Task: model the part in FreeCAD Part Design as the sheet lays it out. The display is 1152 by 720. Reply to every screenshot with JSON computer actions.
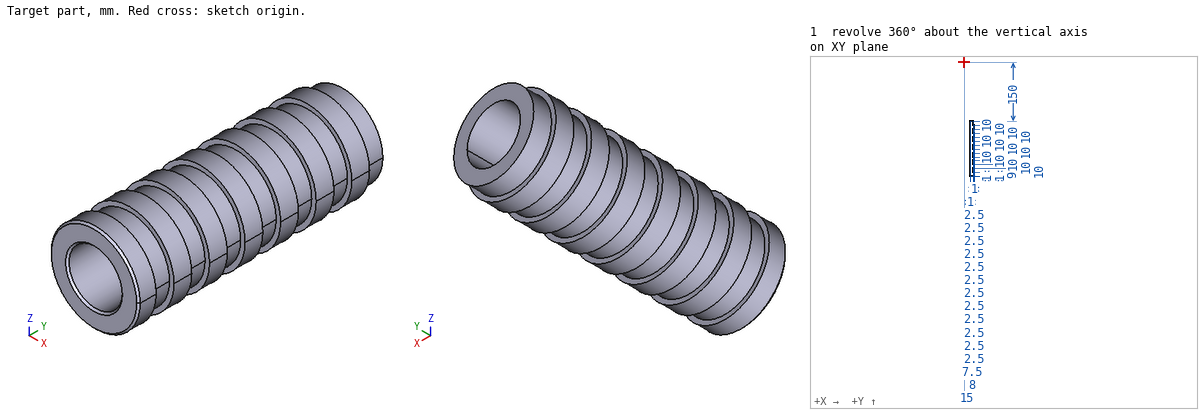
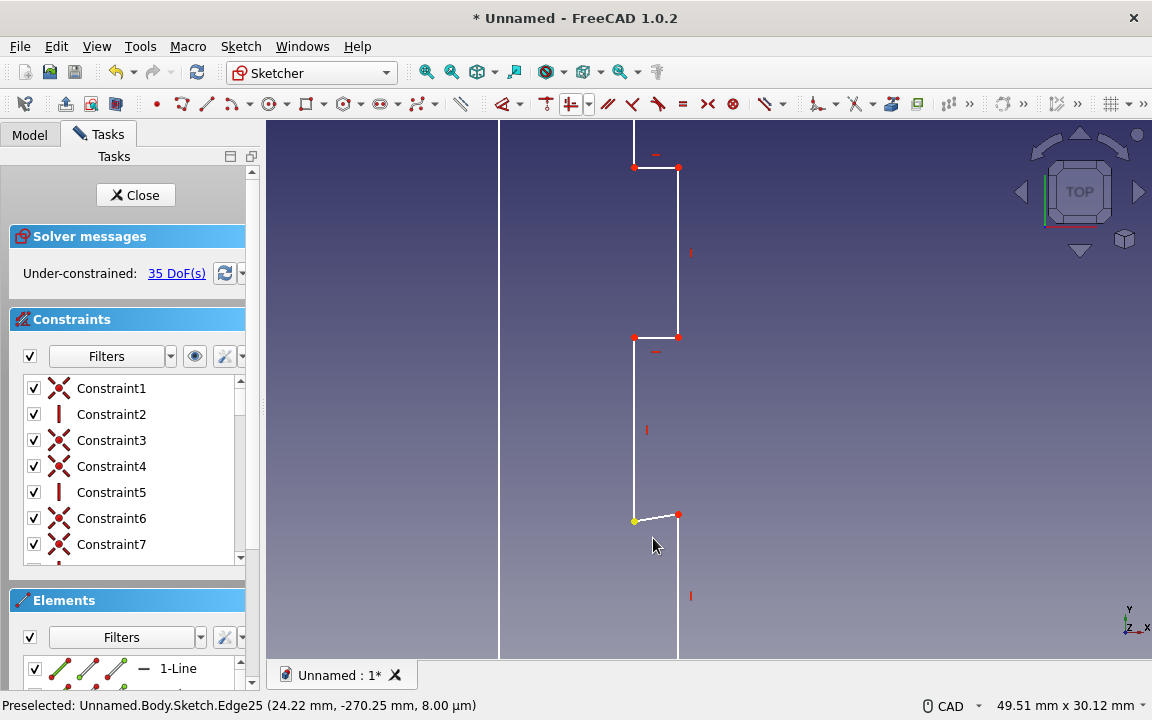
{"action": "left_click", "coordinate": [647, 519]}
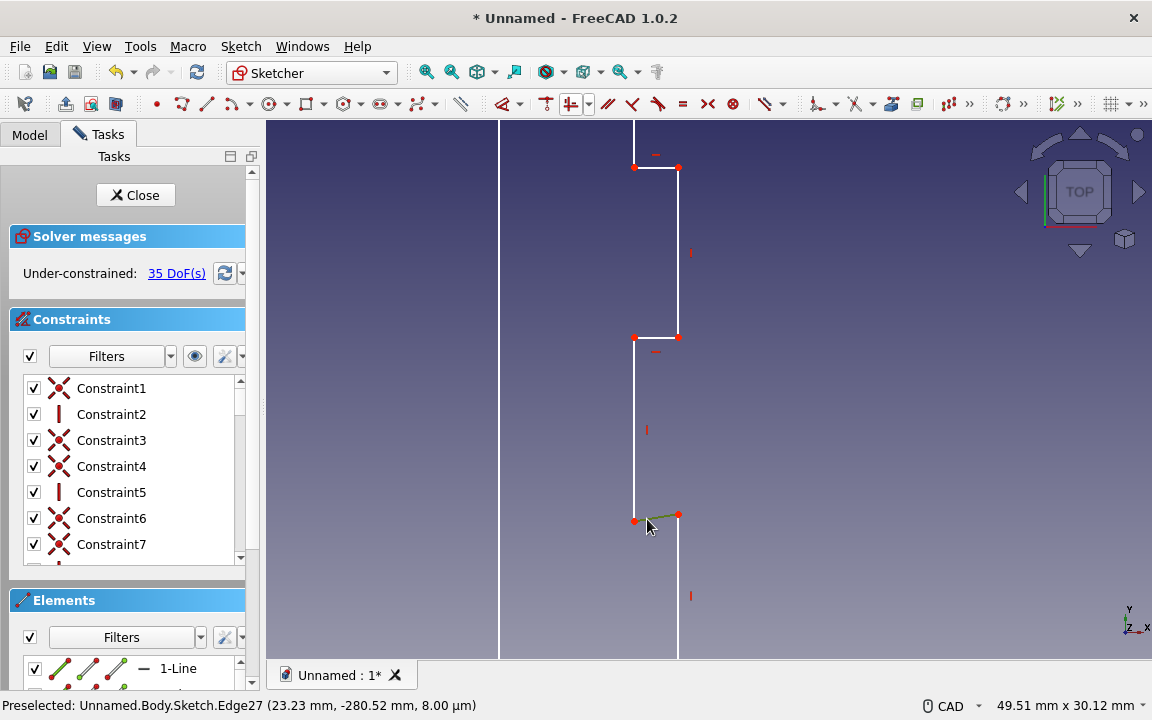
{"action": "key", "text": "h"}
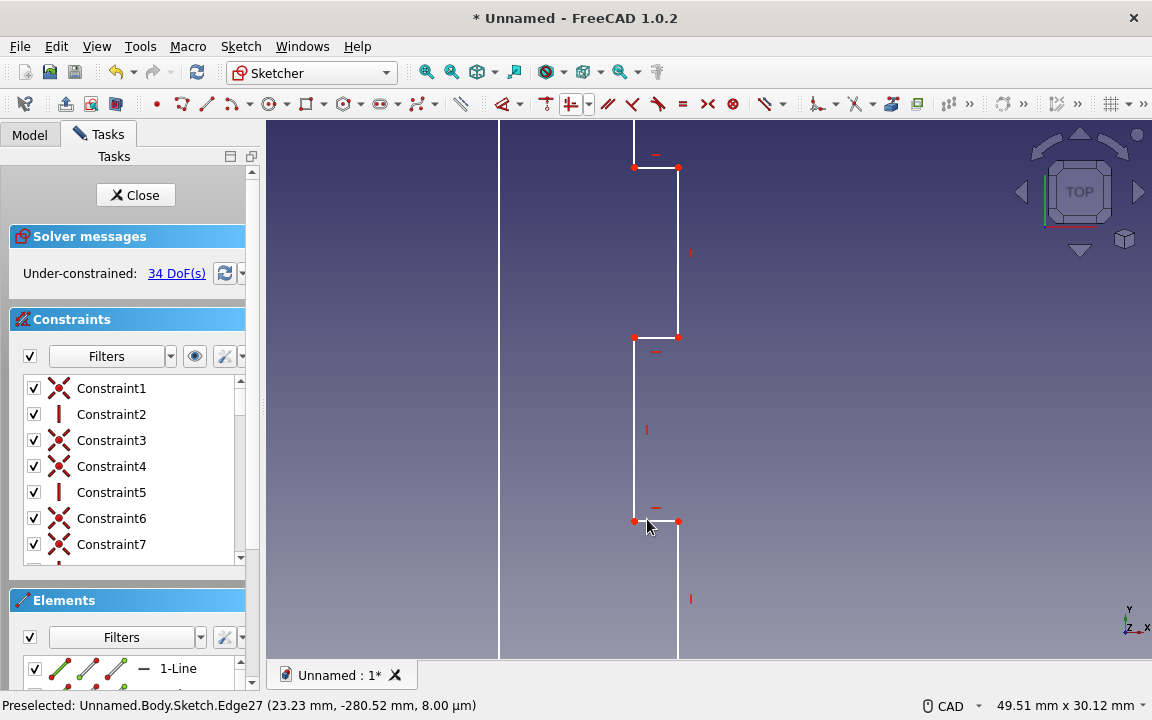
{"action": "key", "text": "d"}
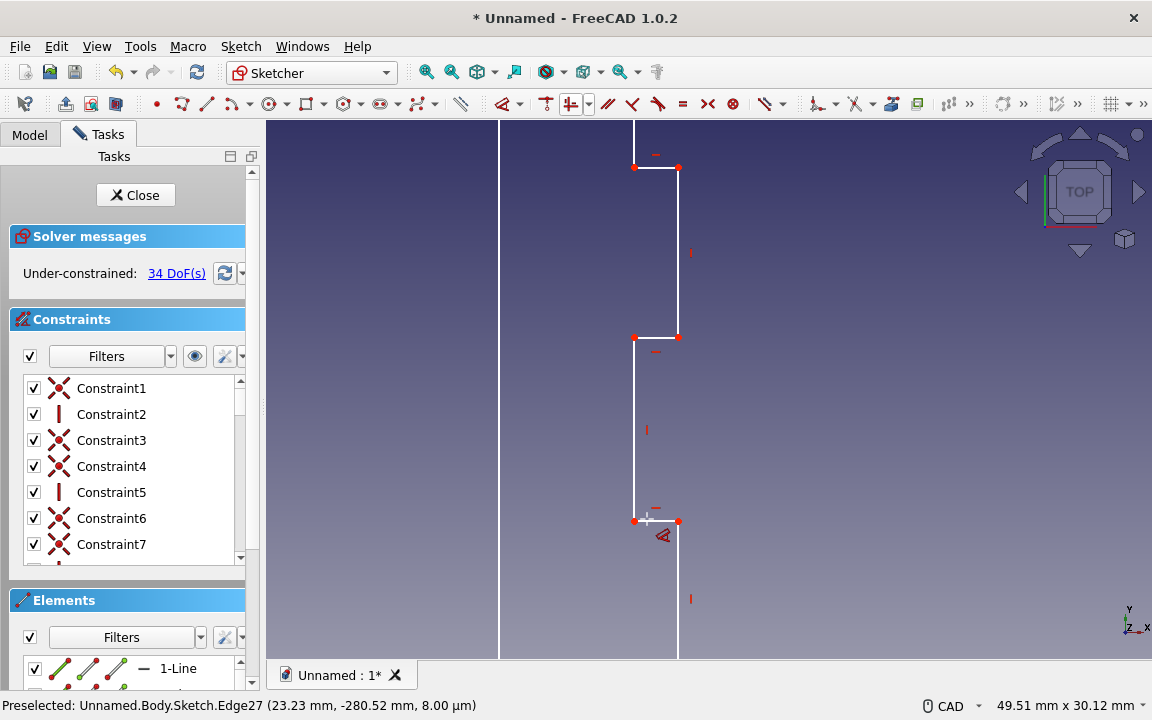
{"action": "scroll", "coordinate": [653, 538], "scroll_direction": "down", "scroll_amount": 14}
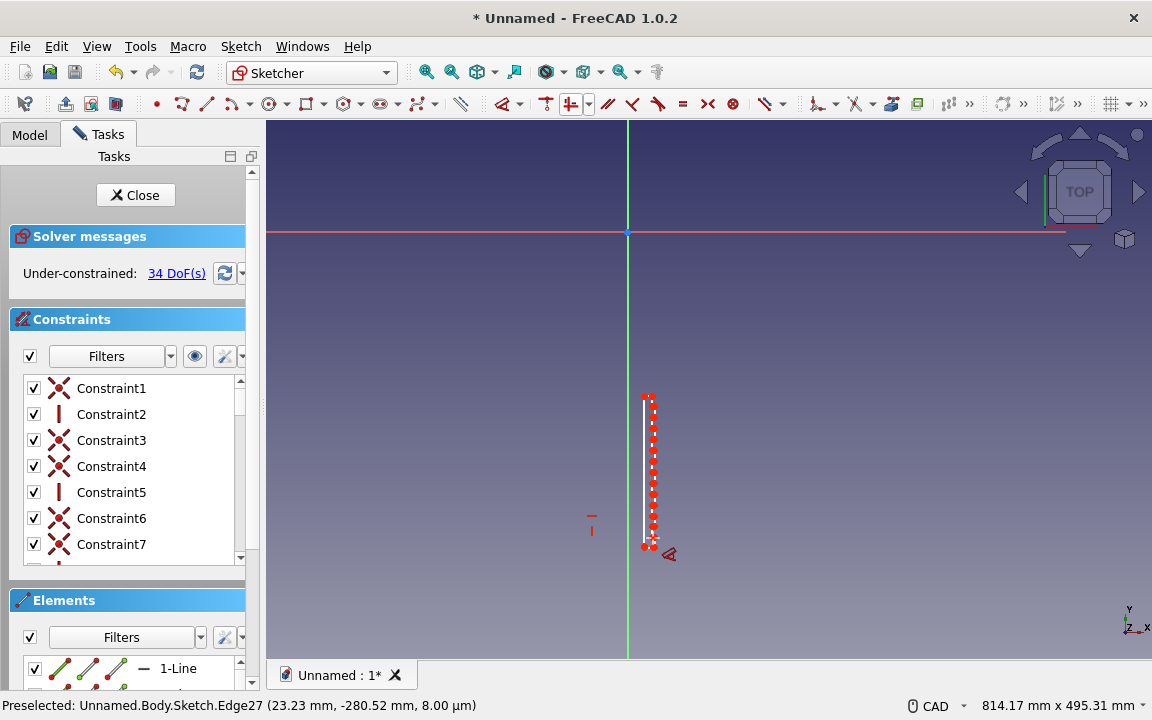
{"action": "scroll", "coordinate": [655, 541], "scroll_direction": "up", "scroll_amount": 8}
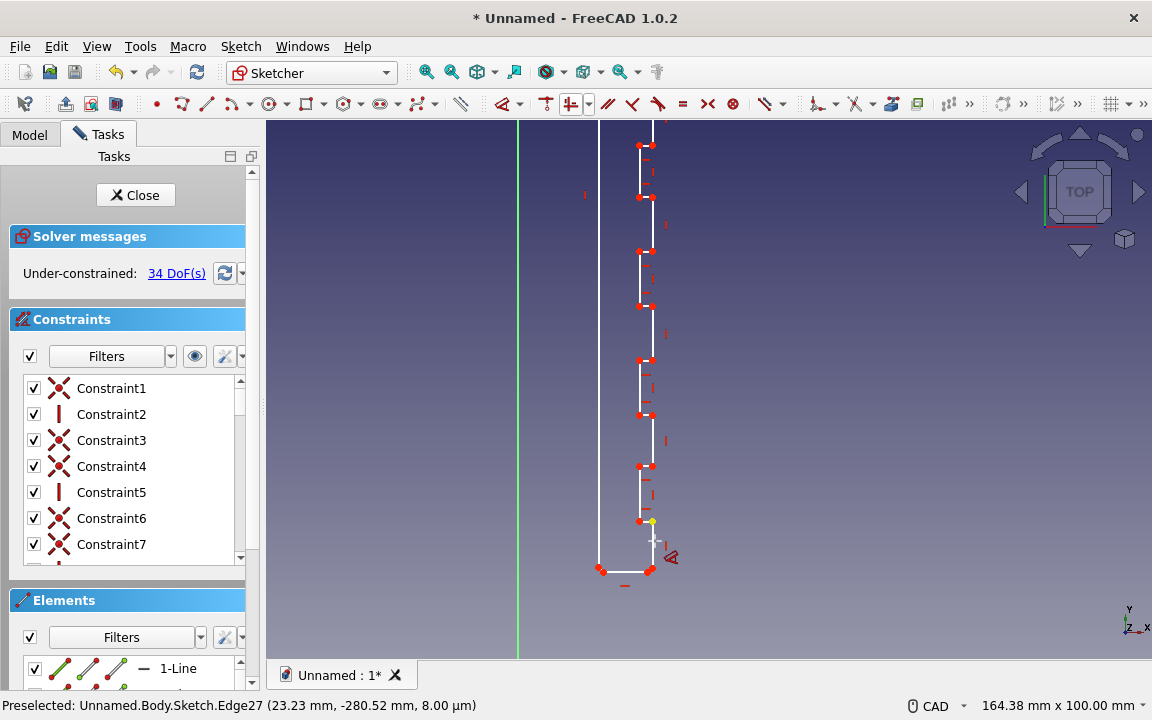
{"action": "left_click", "coordinate": [653, 536]}
{"action": "left_click", "coordinate": [687, 545]}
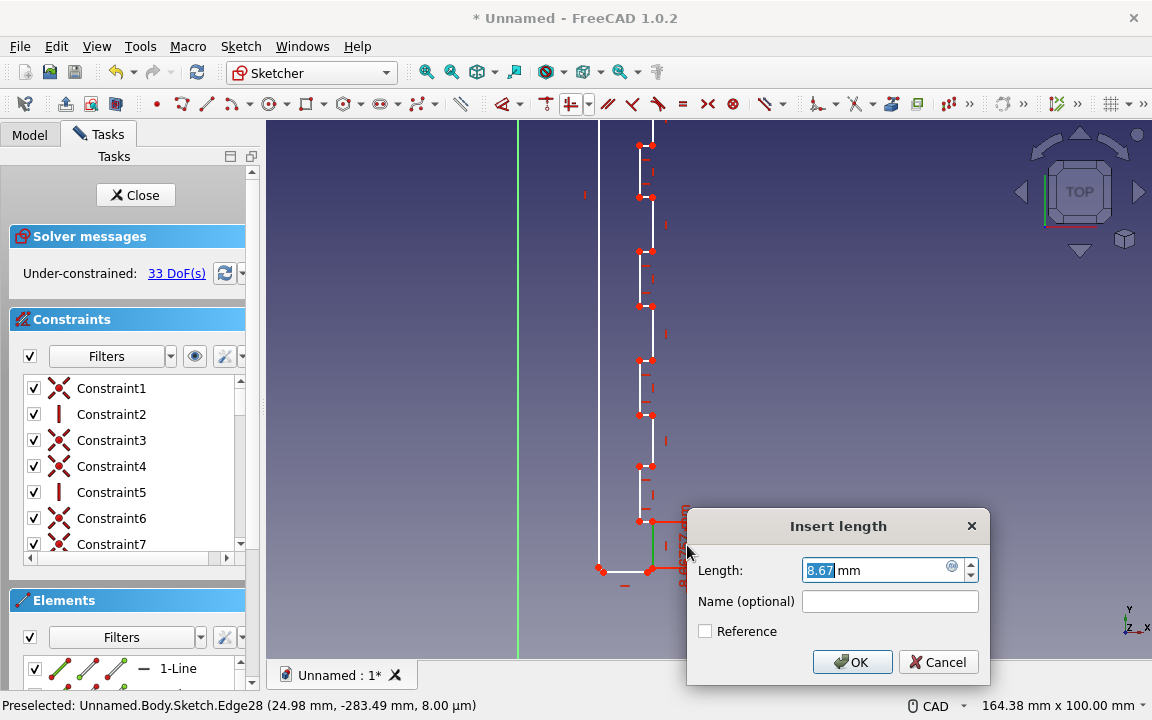
{"action": "type", "text": "9"}
{"action": "key", "text": "Return"}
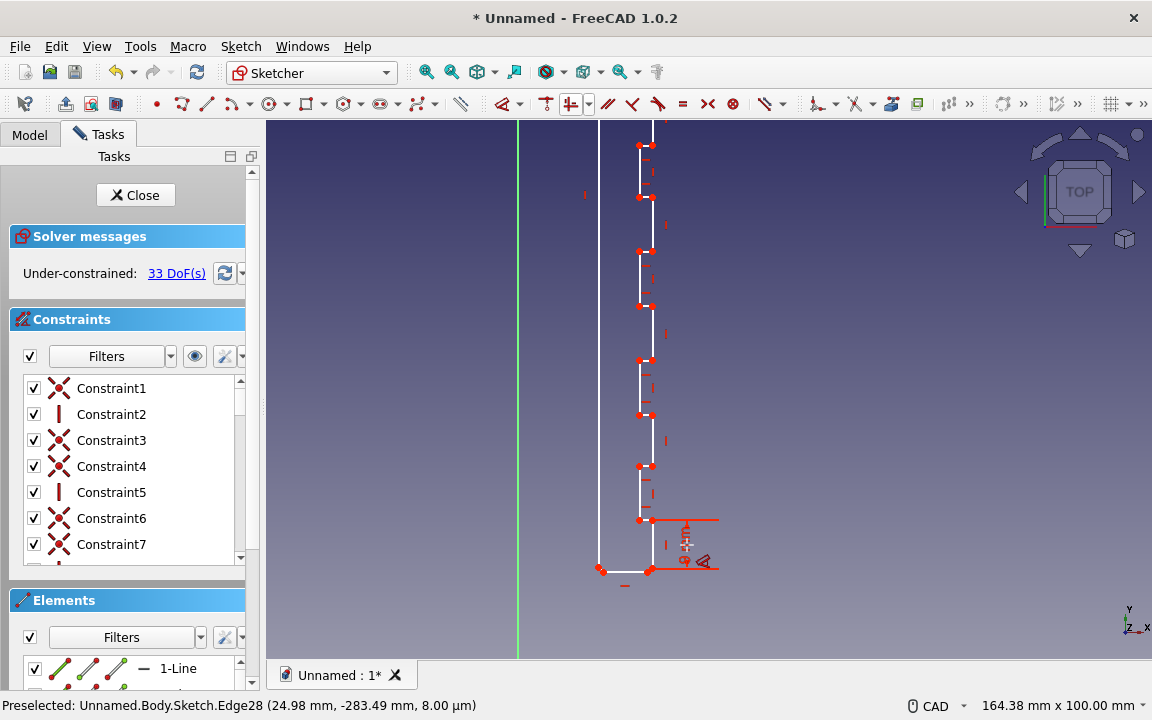
{"action": "left_click", "coordinate": [634, 572]}
{"action": "left_click", "coordinate": [626, 606]}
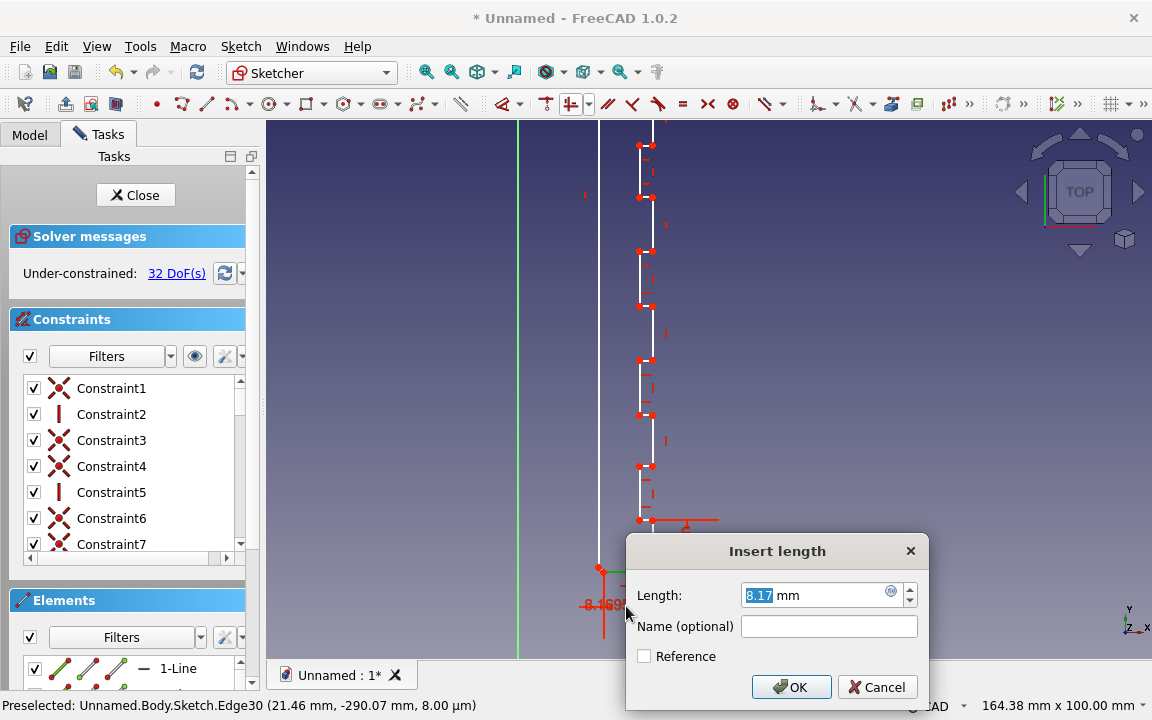
{"action": "type", "text": "8"}
{"action": "key", "text": "Return"}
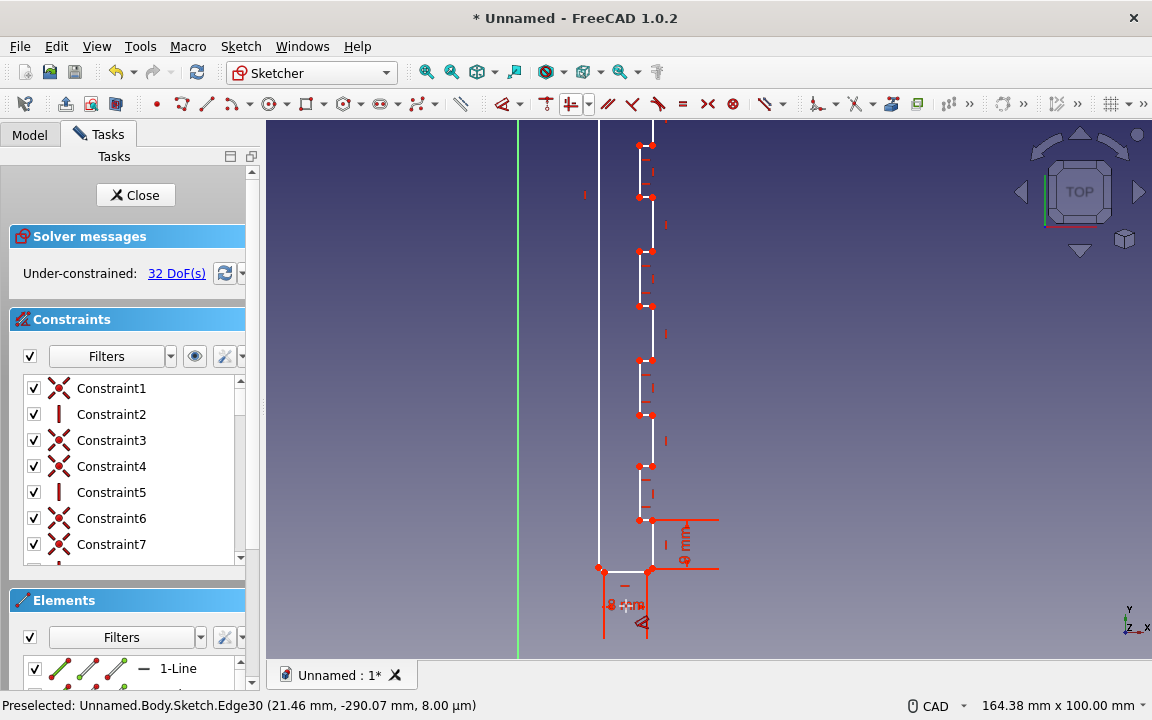
{"action": "scroll", "coordinate": [654, 541], "scroll_direction": "down", "scroll_amount": 8}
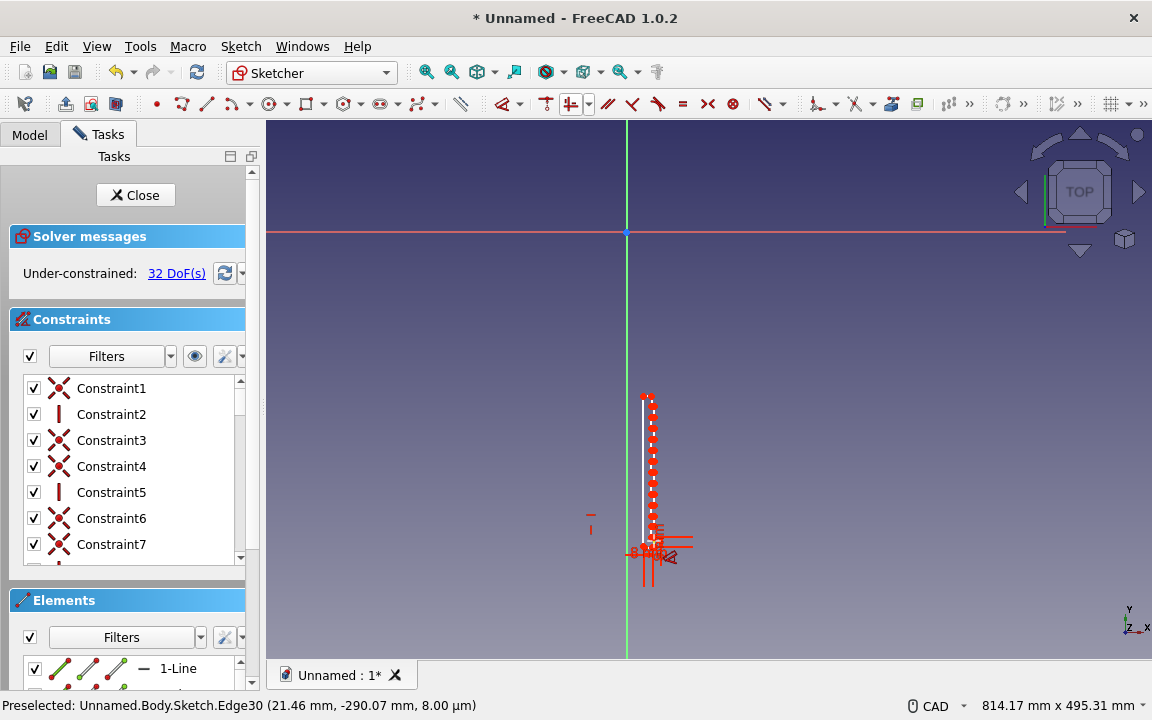
{"action": "scroll", "coordinate": [652, 399], "scroll_direction": "up", "scroll_amount": 8}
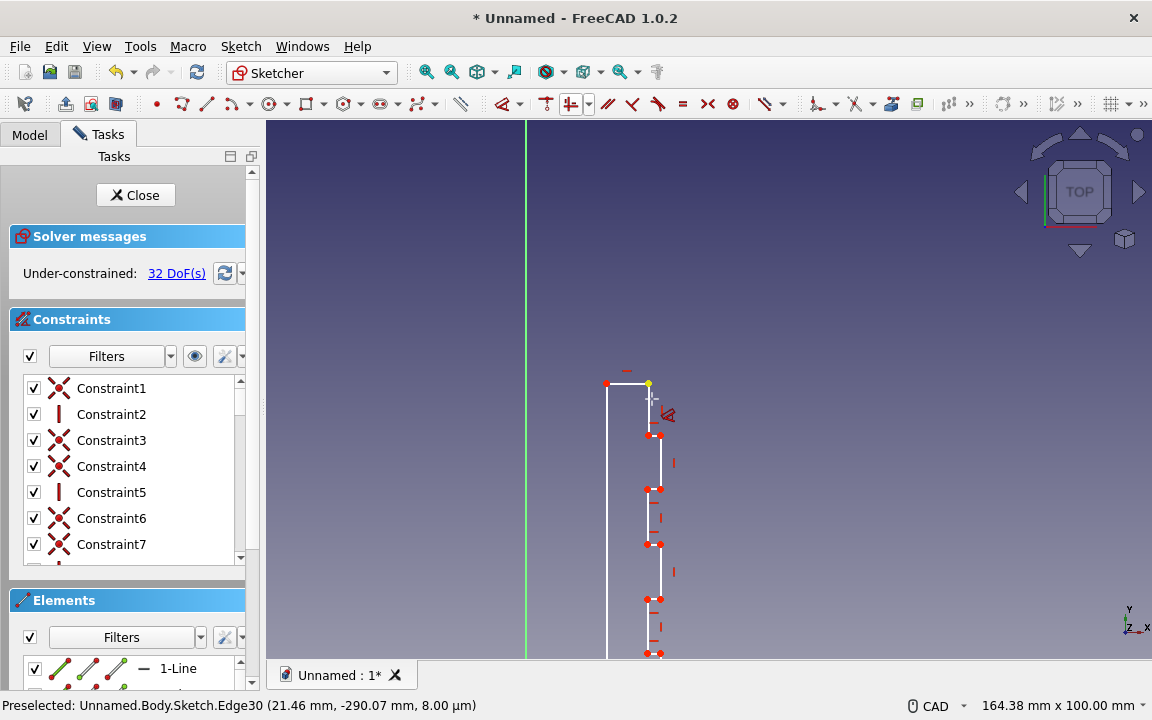
{"action": "left_click", "coordinate": [649, 399]}
{"action": "left_click", "coordinate": [683, 410]}